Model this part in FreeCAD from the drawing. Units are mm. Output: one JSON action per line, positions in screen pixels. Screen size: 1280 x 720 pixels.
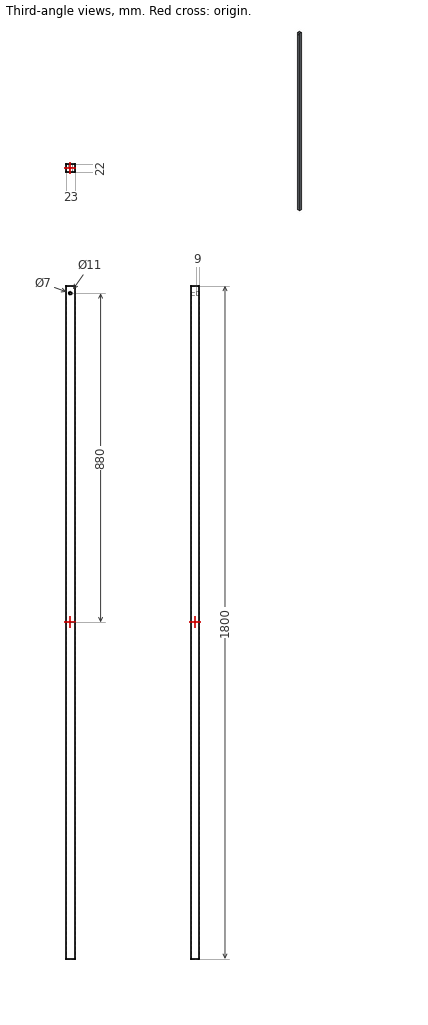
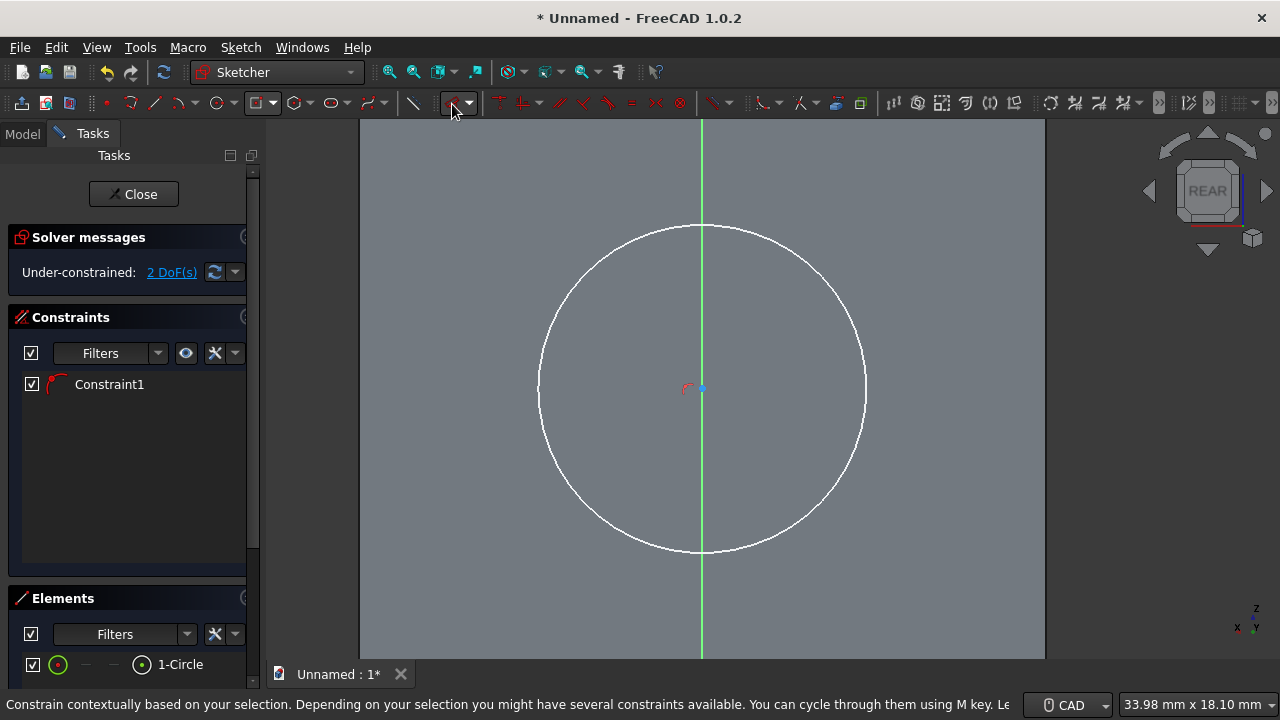
{"action": "left_click", "coordinate": [818, 273]}
{"action": "left_click", "coordinate": [841, 250]}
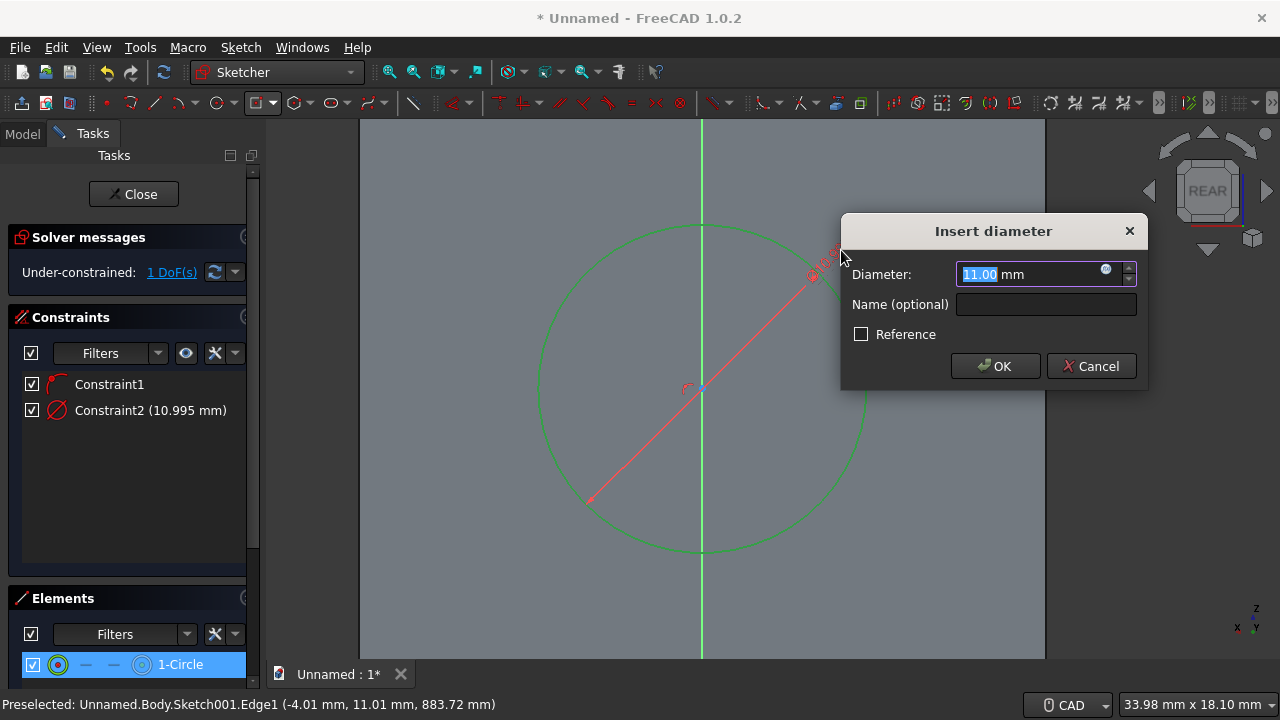
{"action": "type", "text": "11"}
{"action": "key", "text": "Return"}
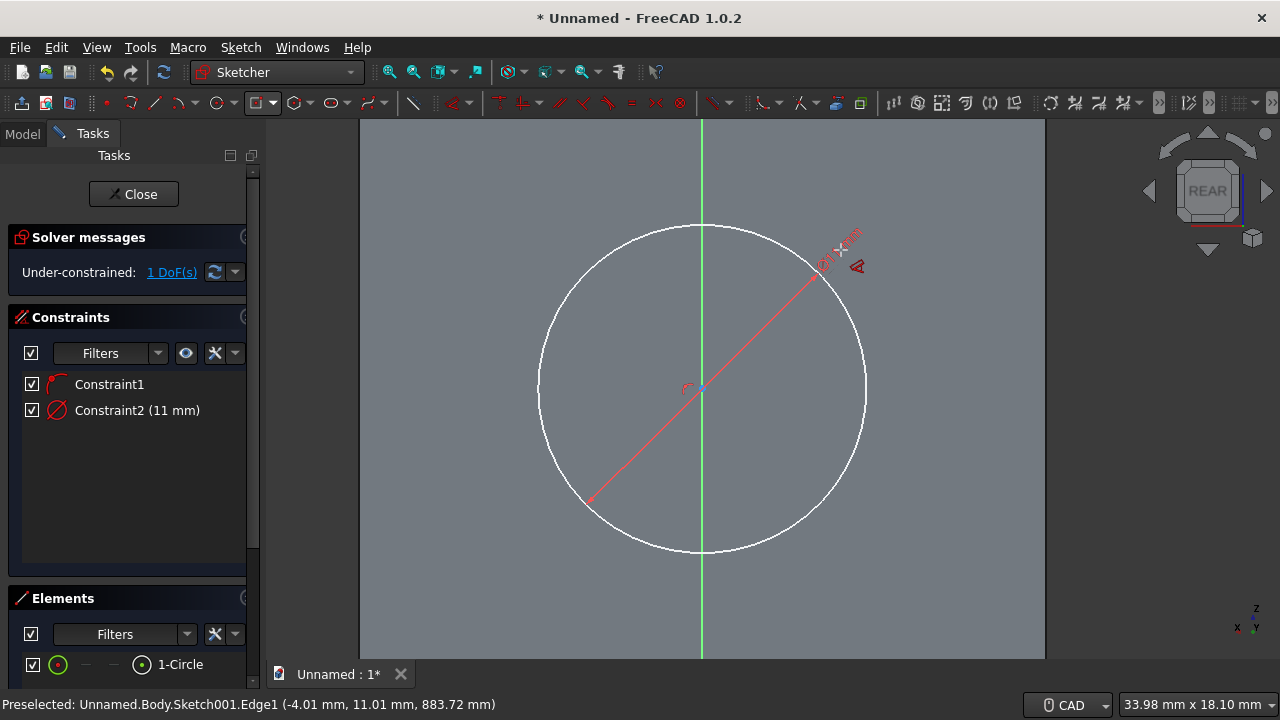
{"action": "left_click", "coordinate": [702, 389]}
{"action": "left_click", "coordinate": [736, 510]}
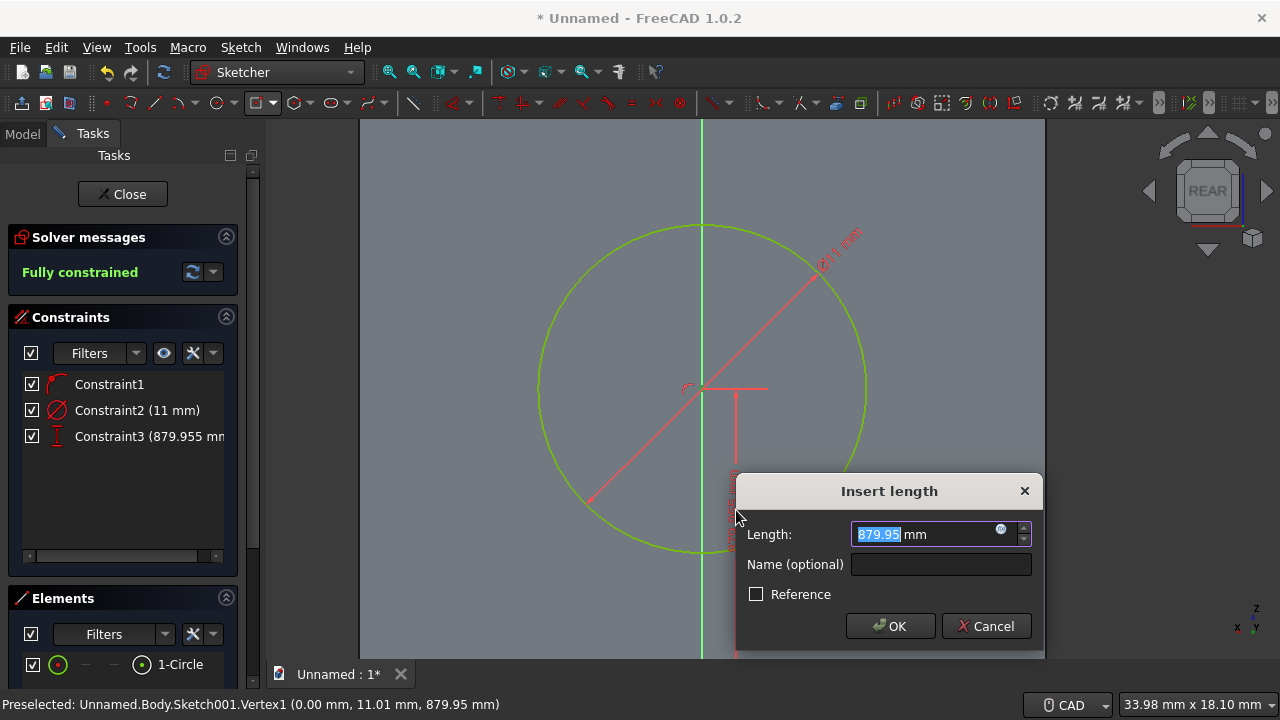
{"action": "type", "text": "880"}
{"action": "key", "text": "Return"}
{"action": "key", "text": "Escape"}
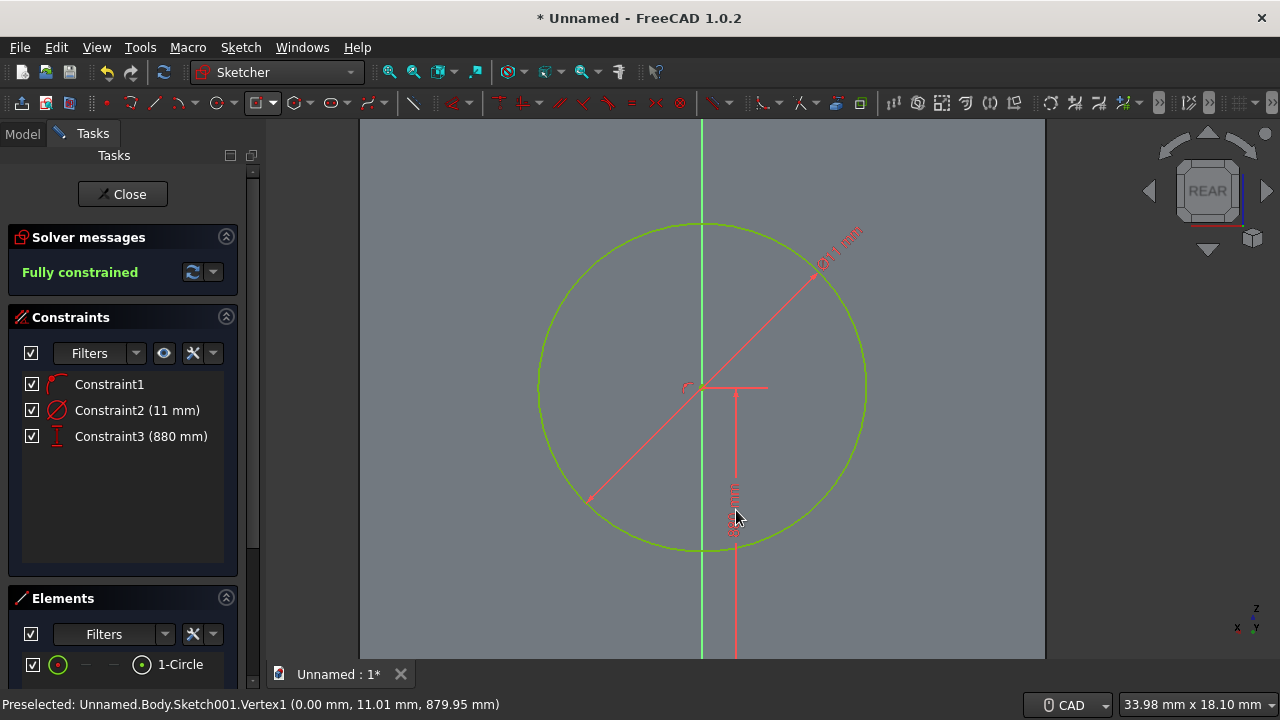
{"action": "left_click", "coordinate": [123, 194]}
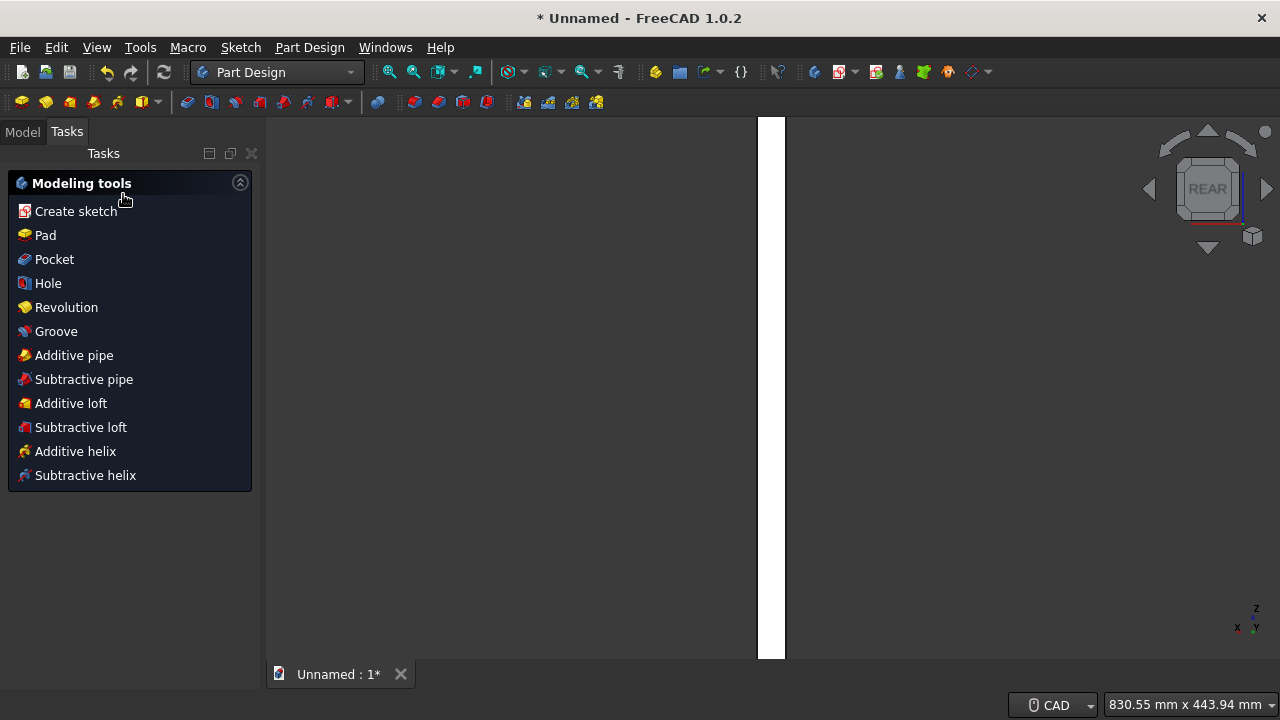
{"action": "left_click", "coordinate": [188, 102]}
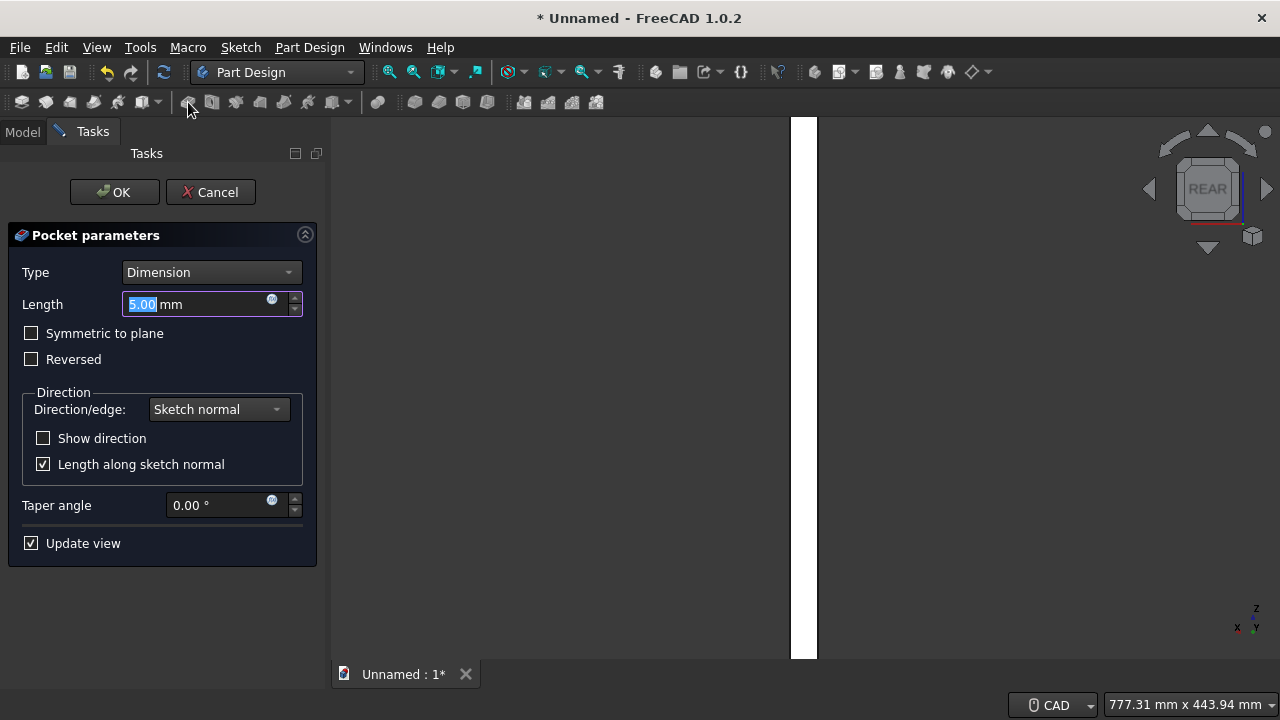
{"action": "type", "text": "9"}
{"action": "key", "text": "Tab"}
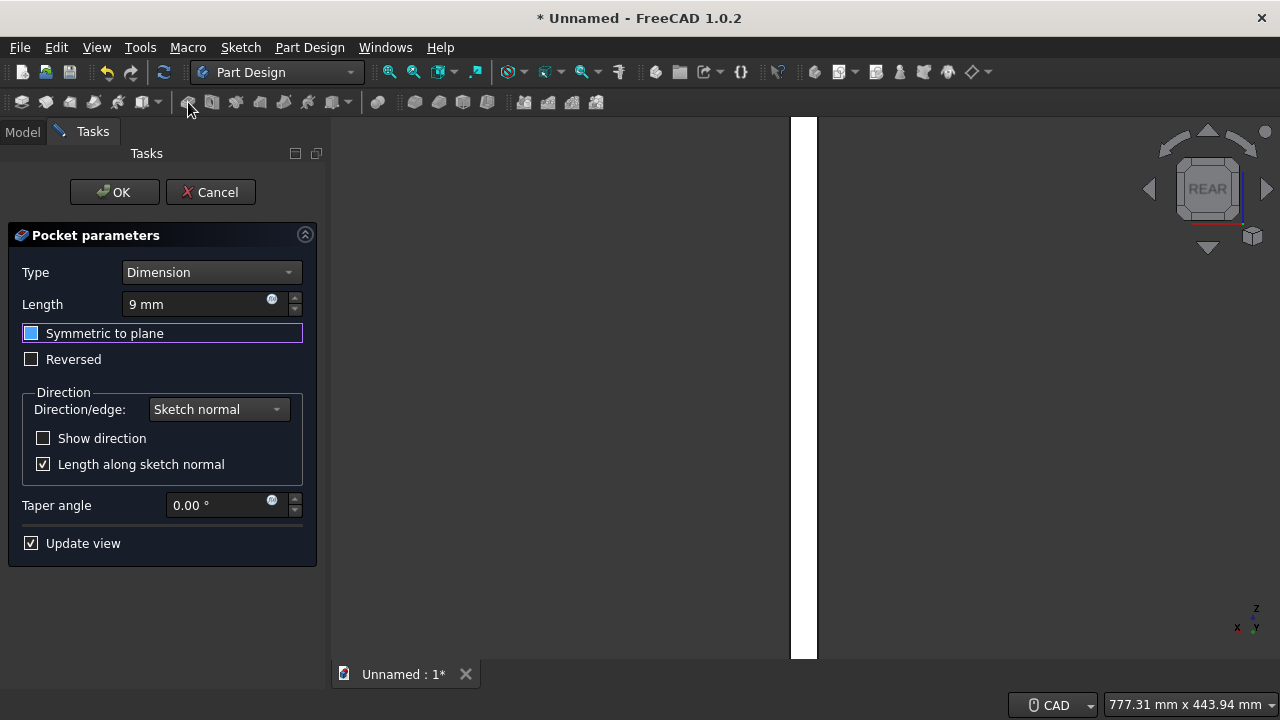
{"action": "left_click", "coordinate": [115, 192]}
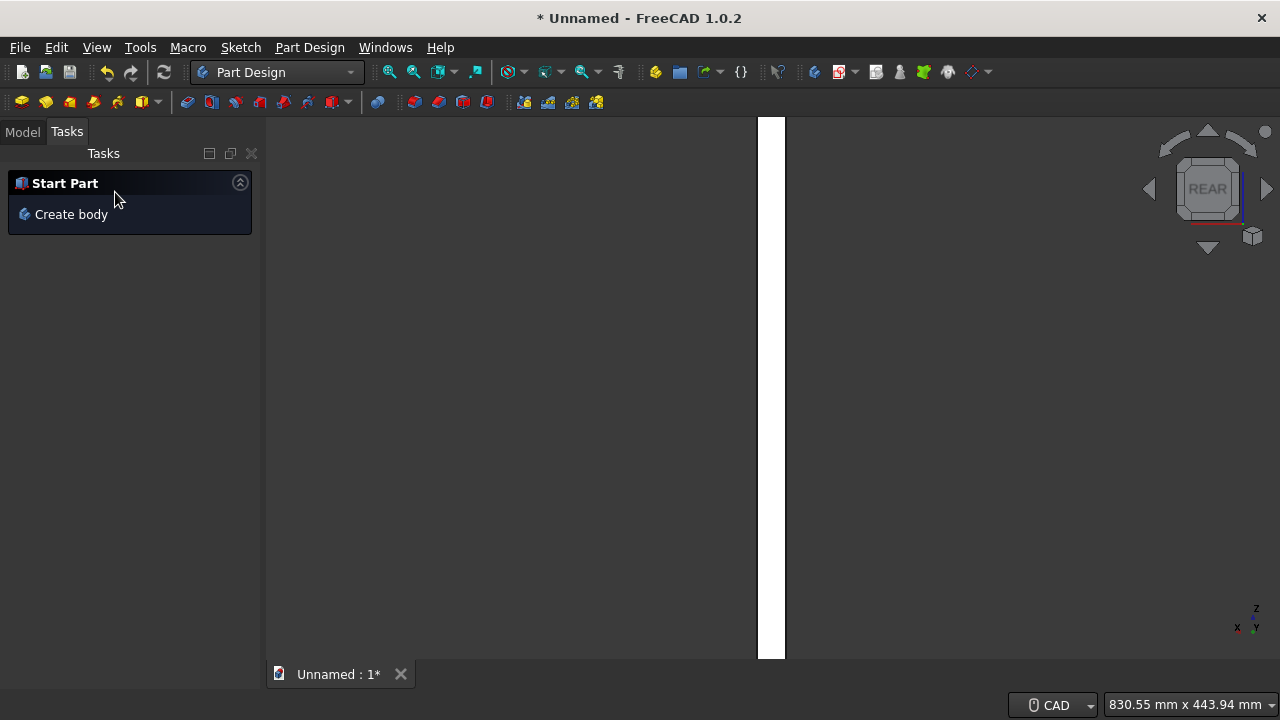
{"action": "left_click", "coordinate": [390, 72]}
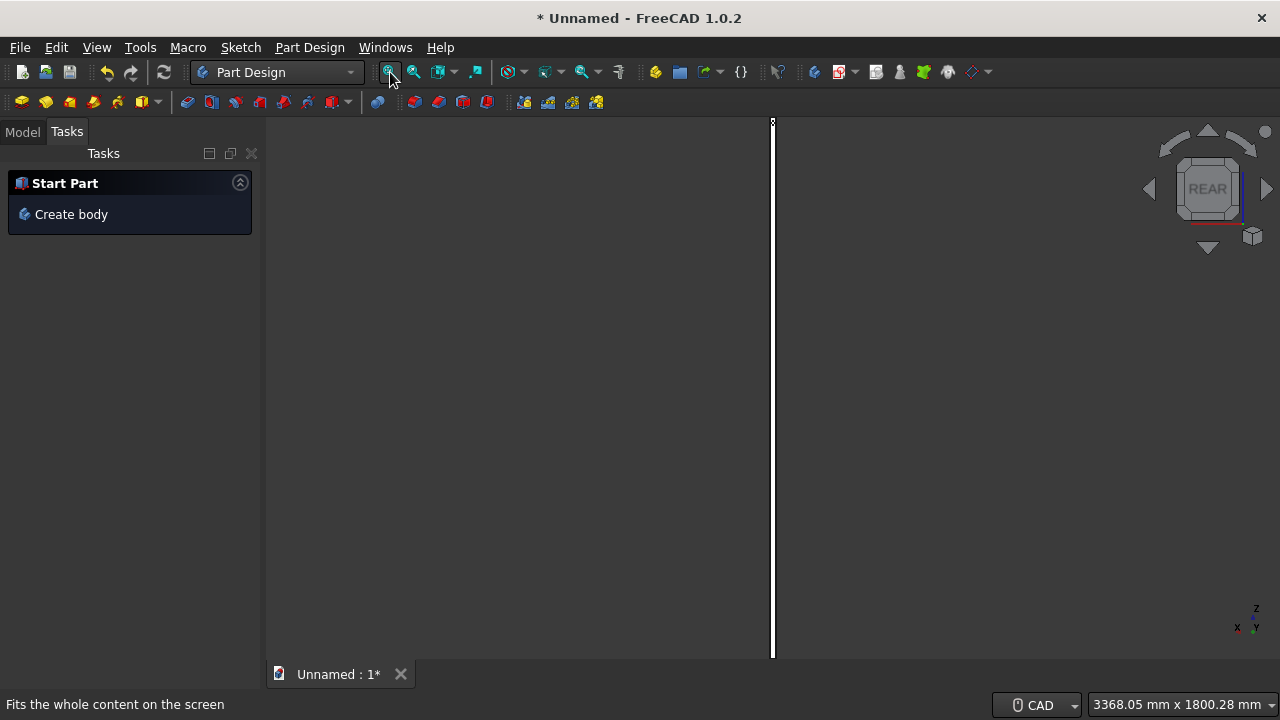
{"action": "key", "text": "5"}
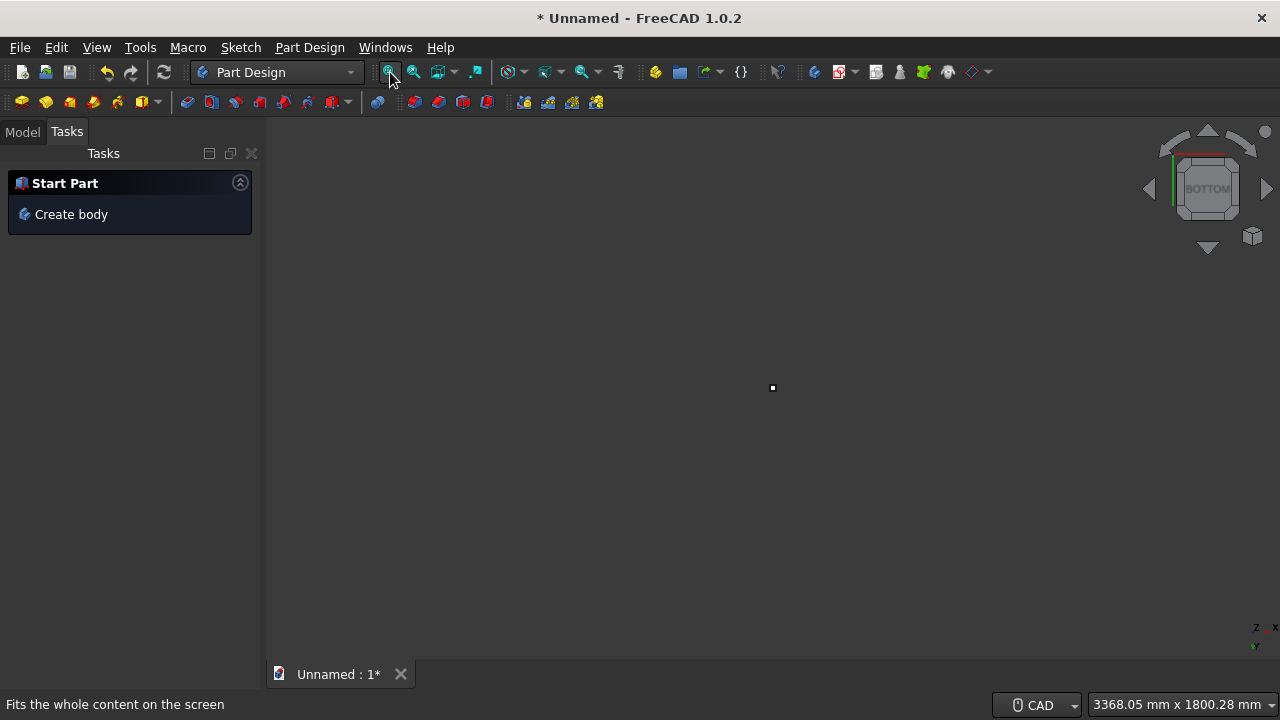
{"action": "left_click", "coordinate": [390, 72]}